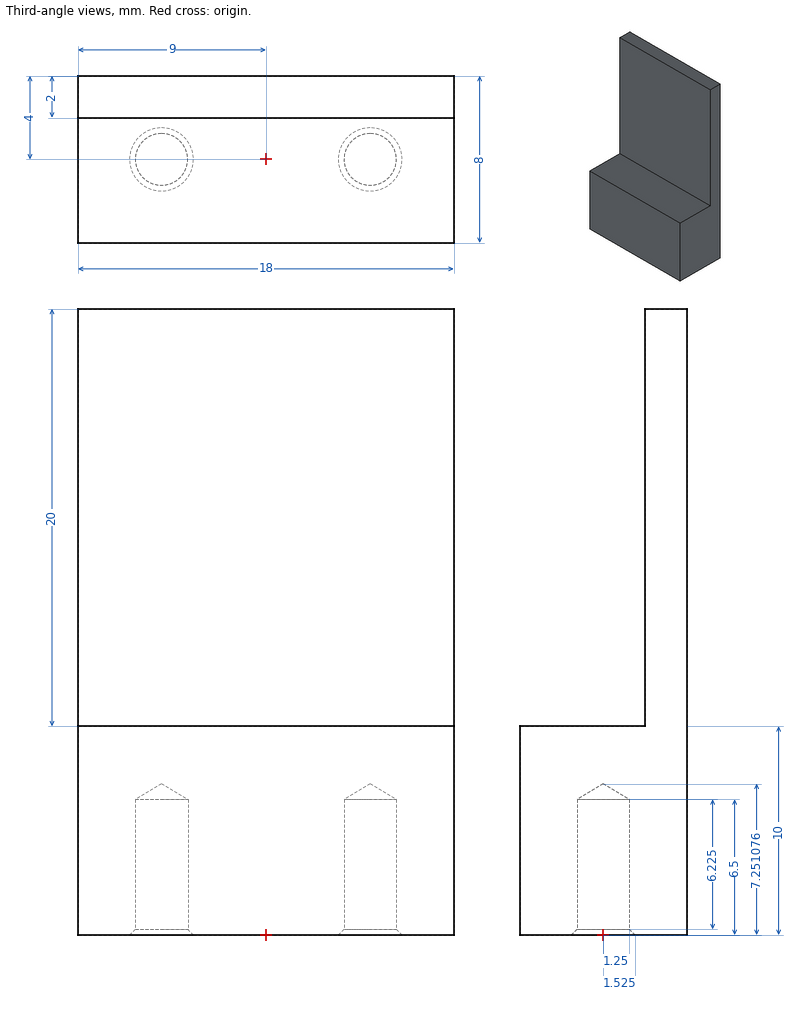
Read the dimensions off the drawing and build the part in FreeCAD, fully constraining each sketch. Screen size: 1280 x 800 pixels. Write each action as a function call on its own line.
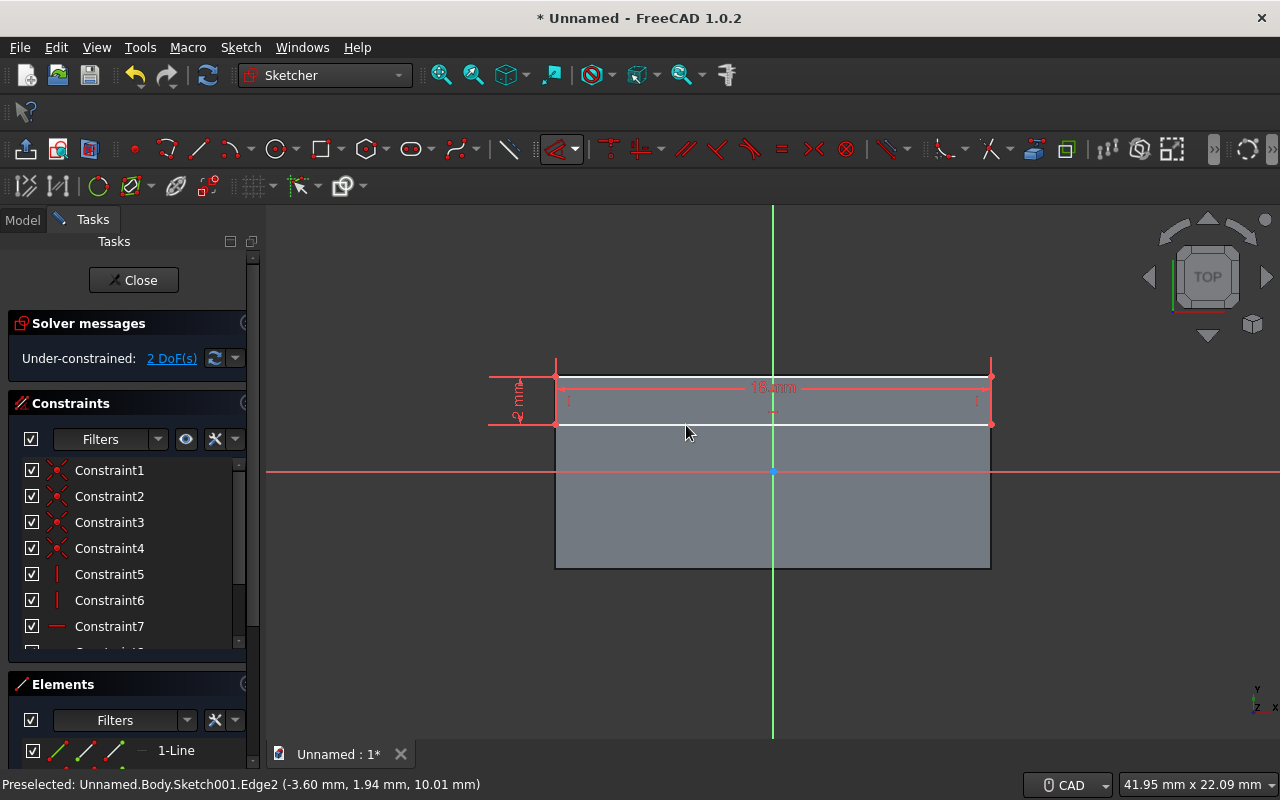
click(556, 377)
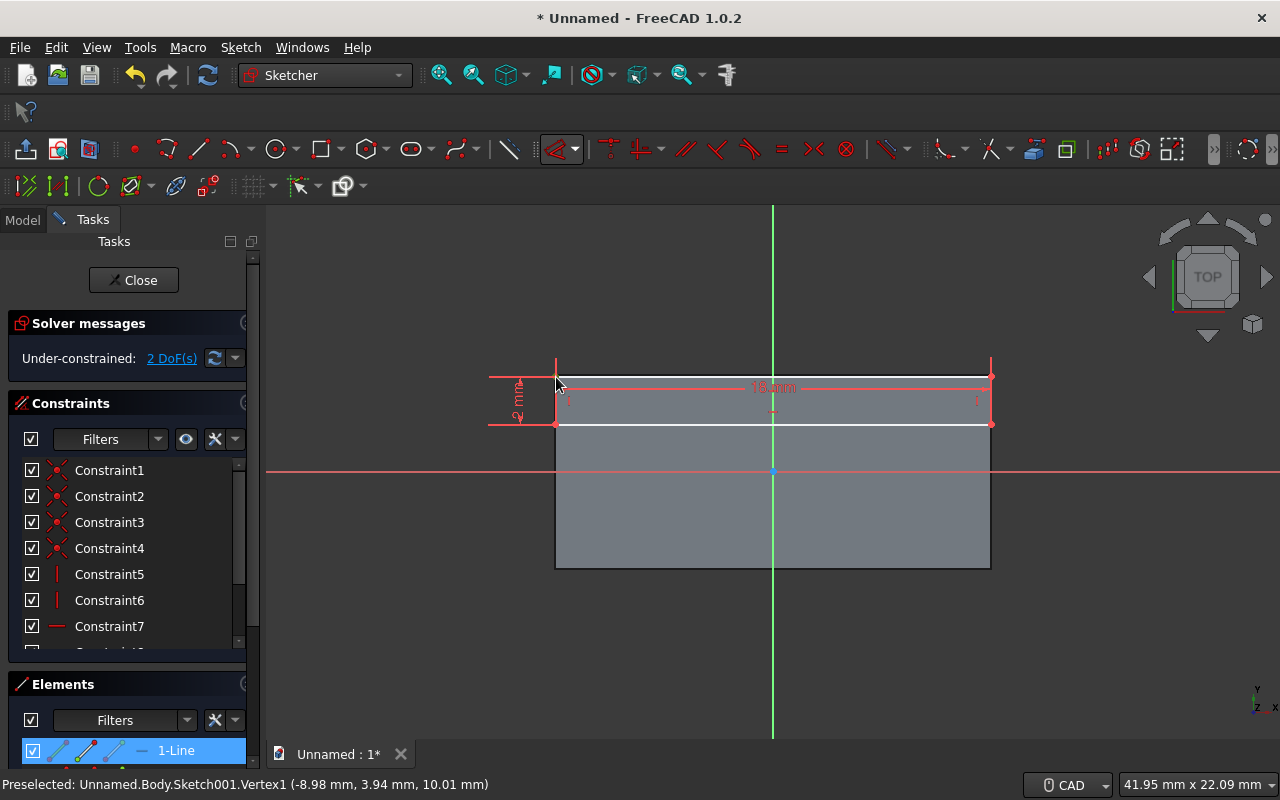
key(l)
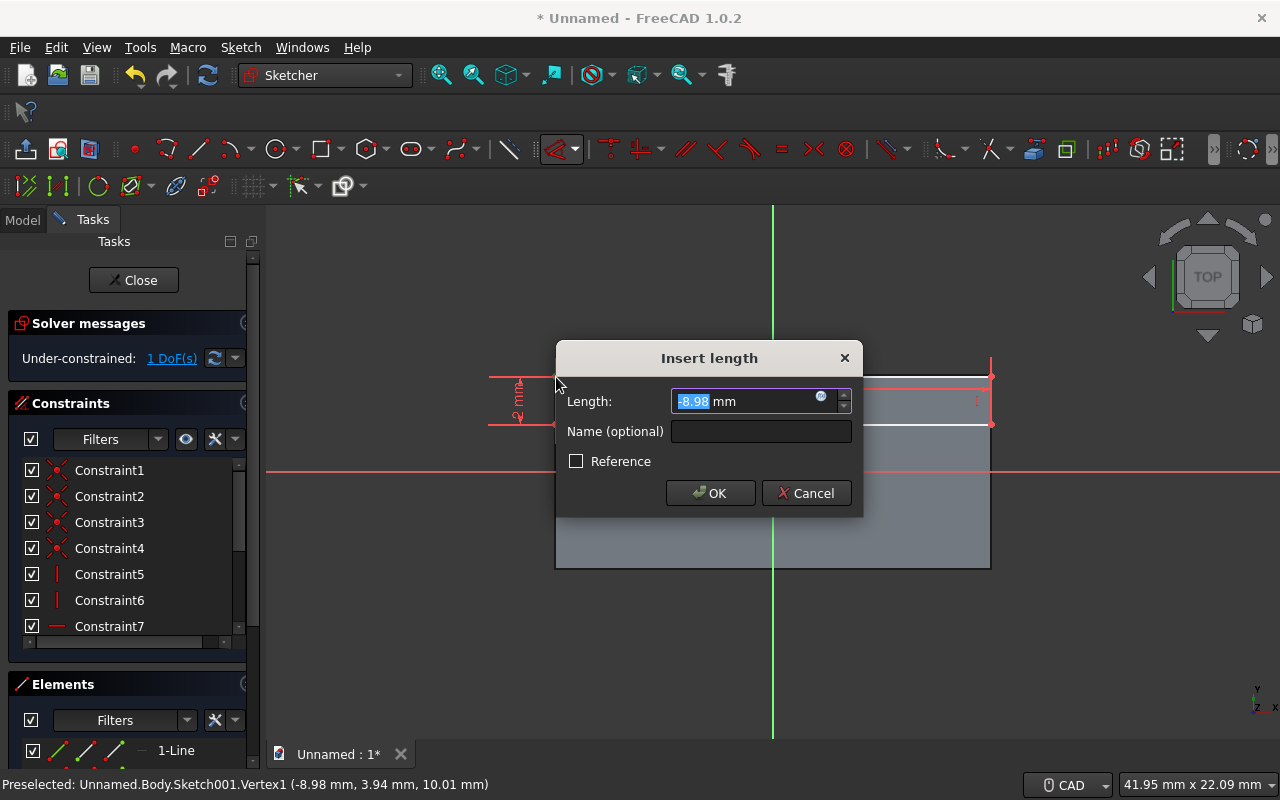
text(-9)
key(Return)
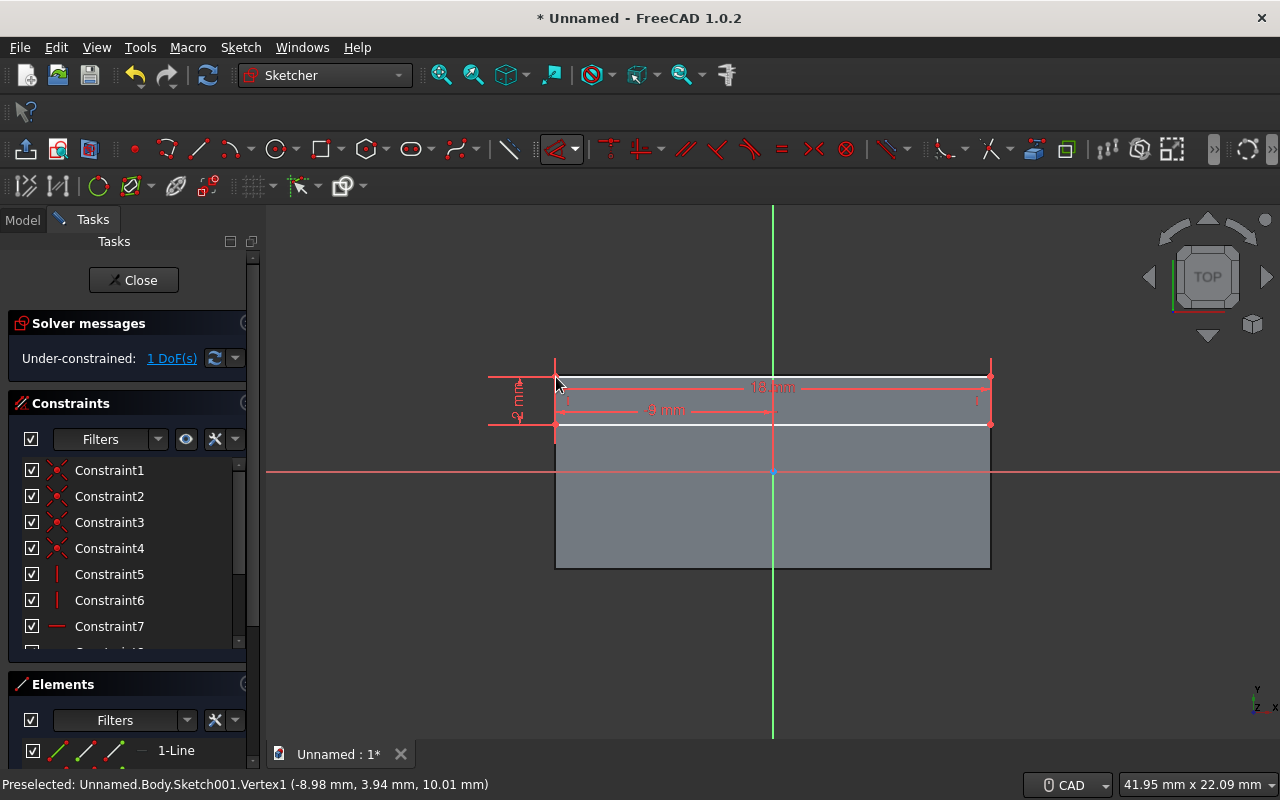
click(555, 377)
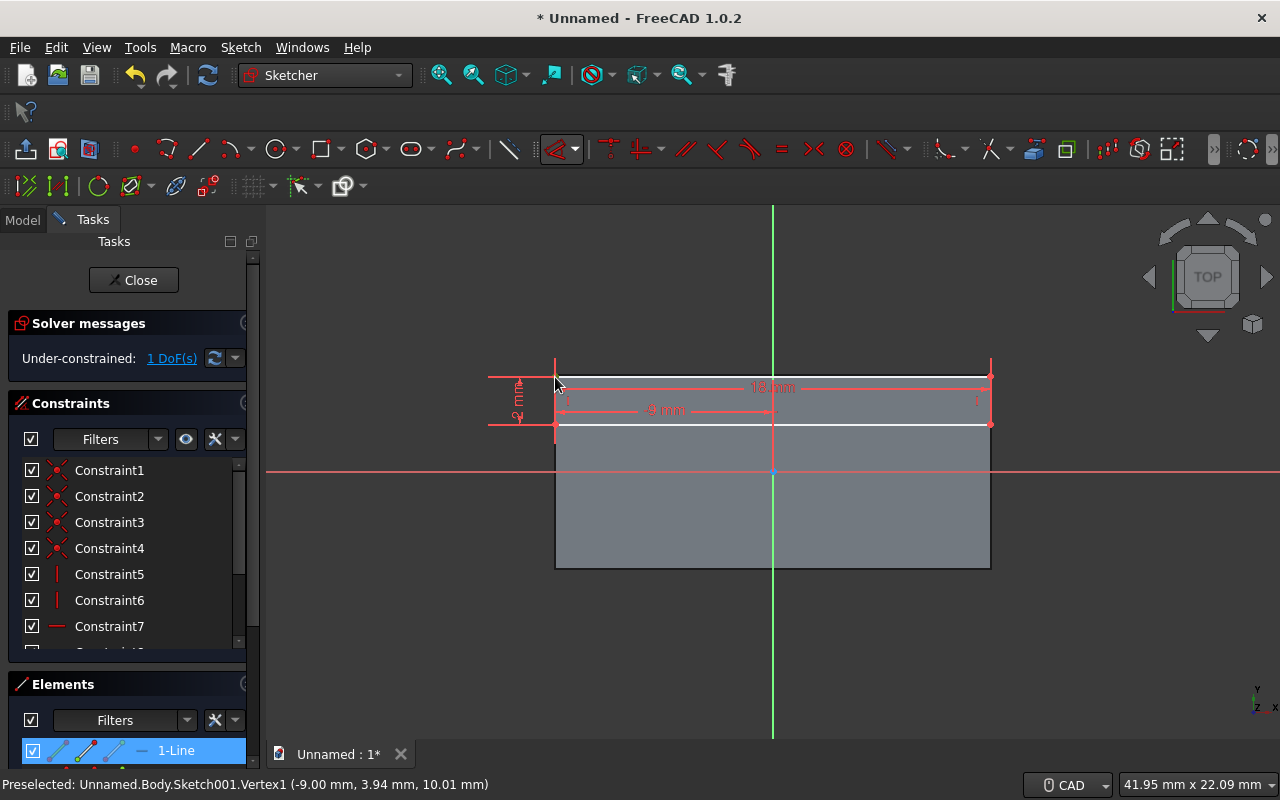
click(578, 150)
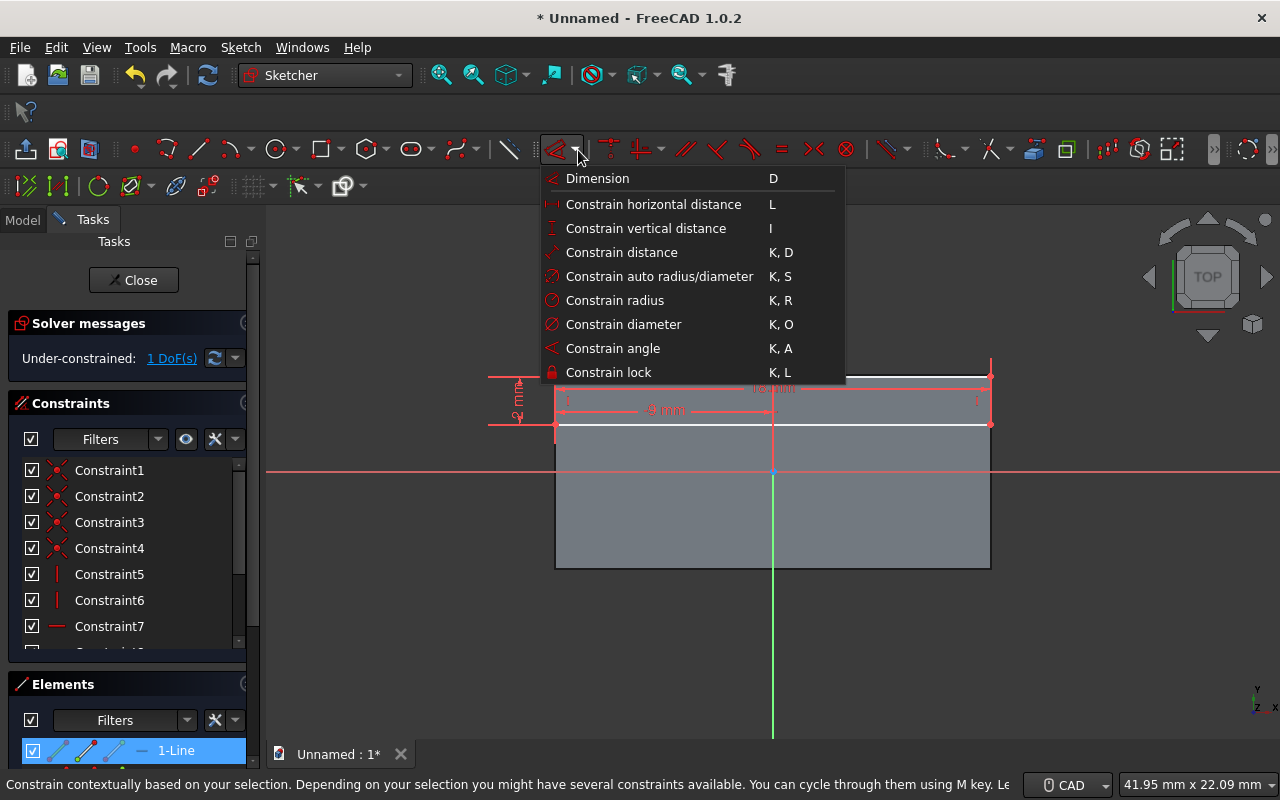
click(693, 228)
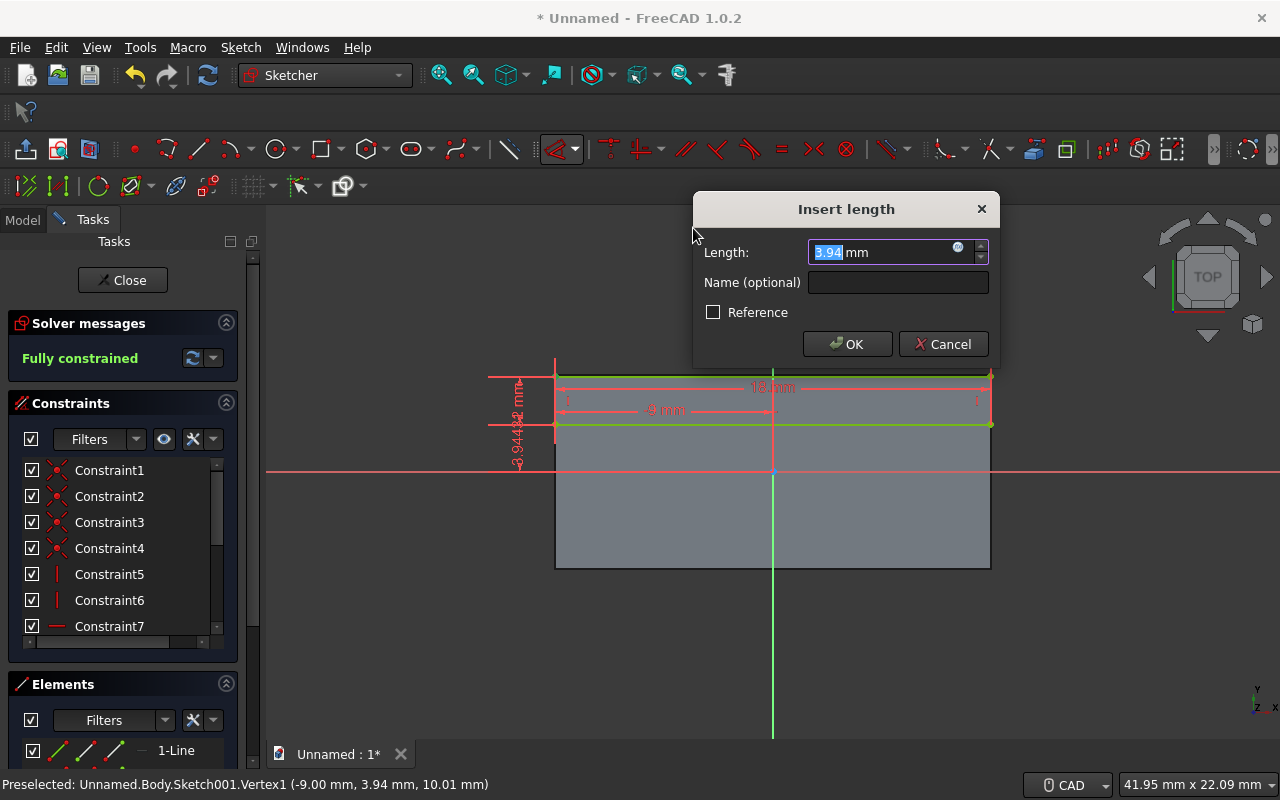
text(4)
key(Return)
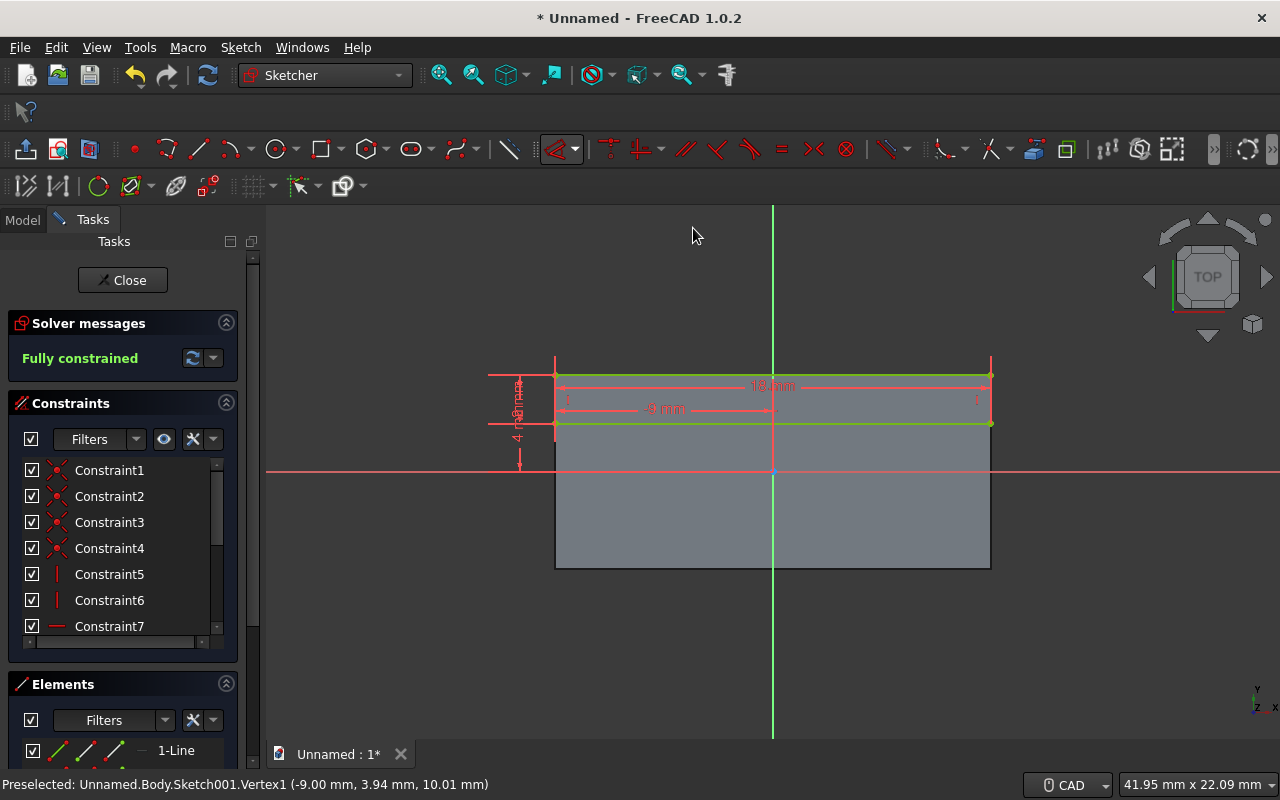
click(123, 280)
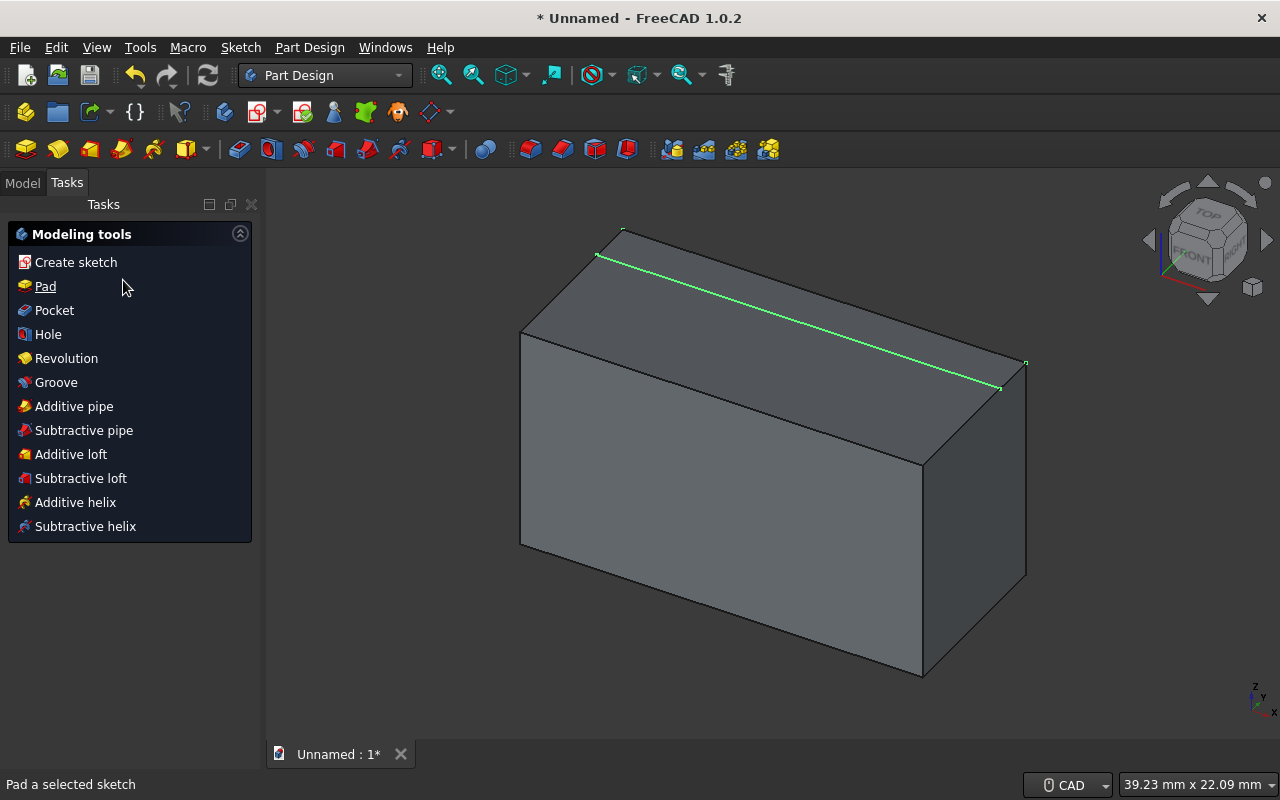
click(26, 150)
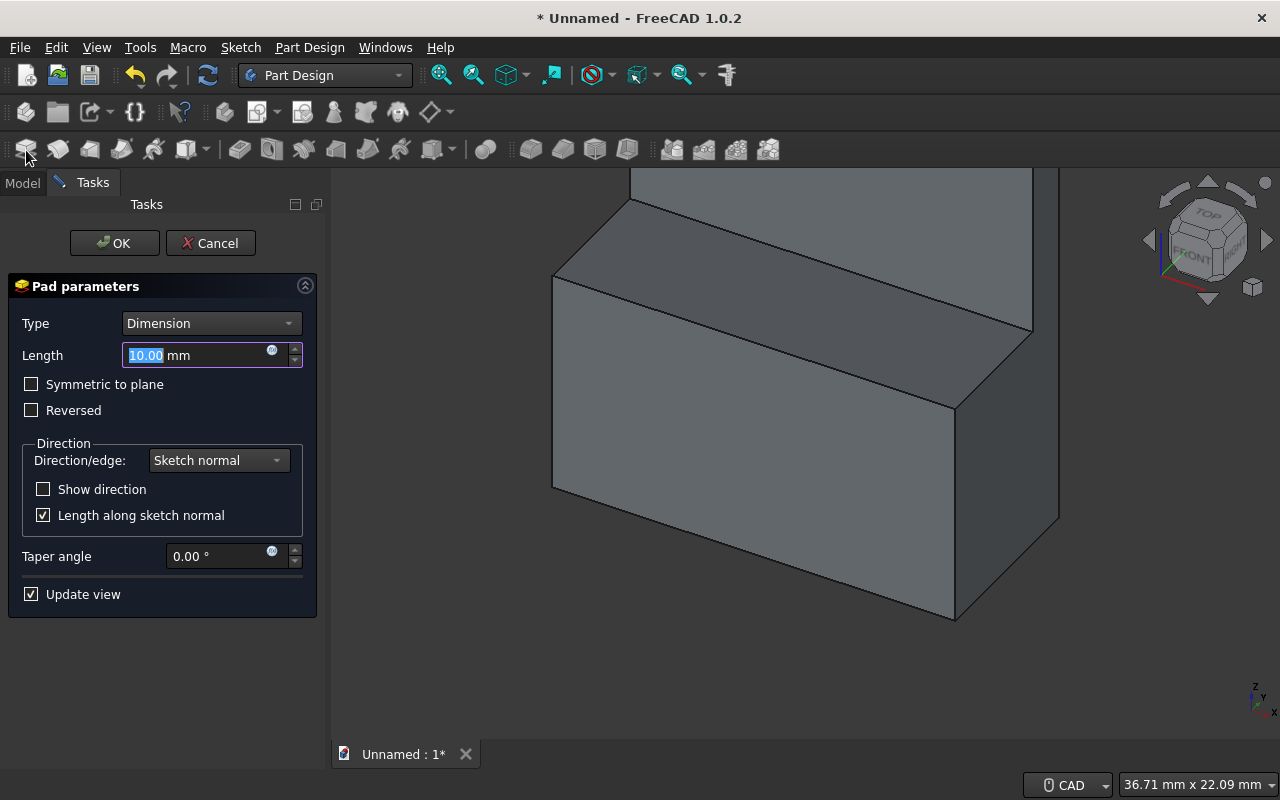
text(20)
key(Tab)